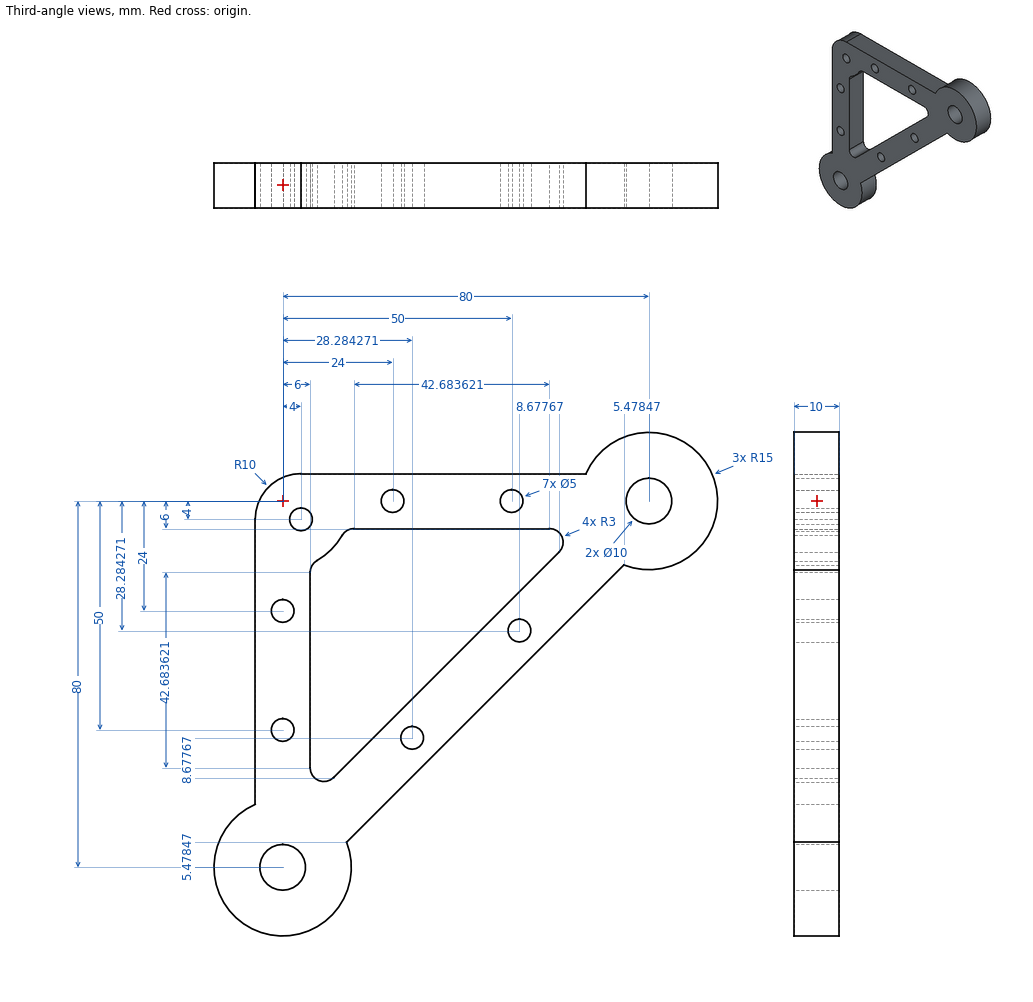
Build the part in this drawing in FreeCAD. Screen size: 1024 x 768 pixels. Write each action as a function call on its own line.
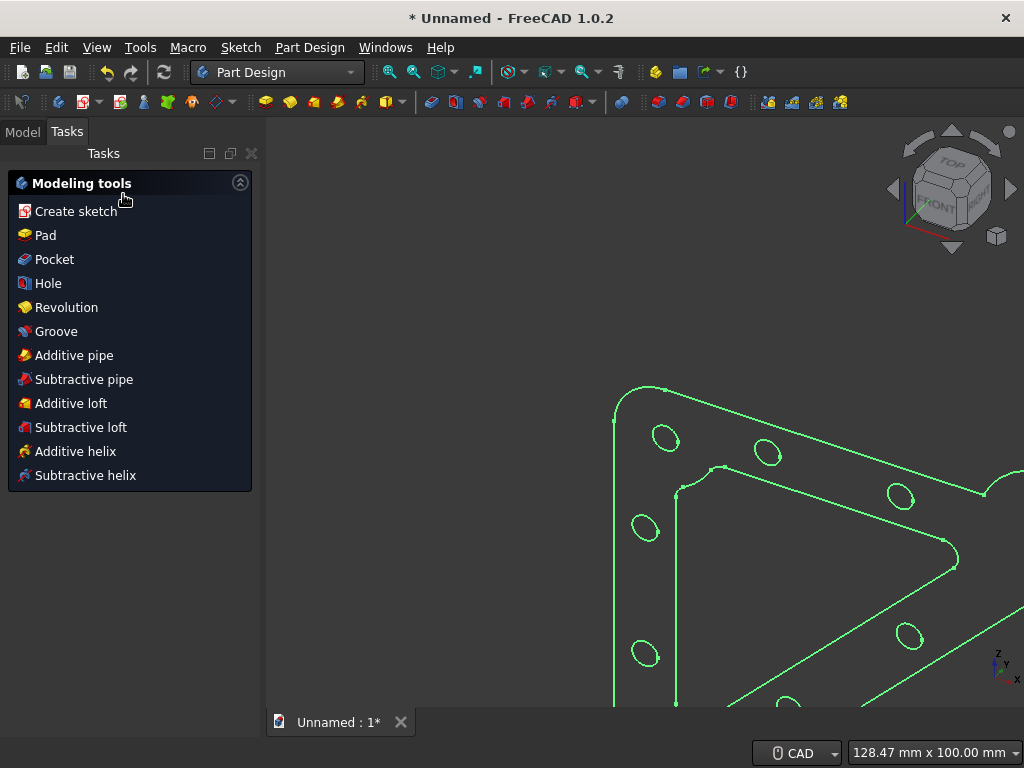
click(266, 102)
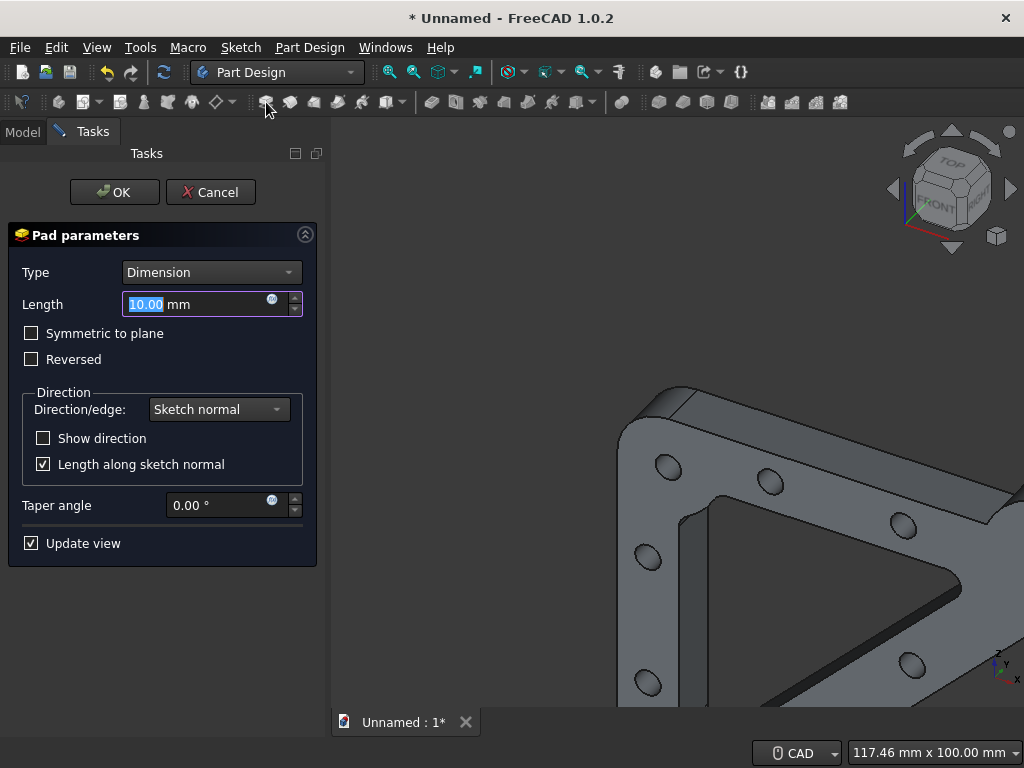
text(10)
key(Tab)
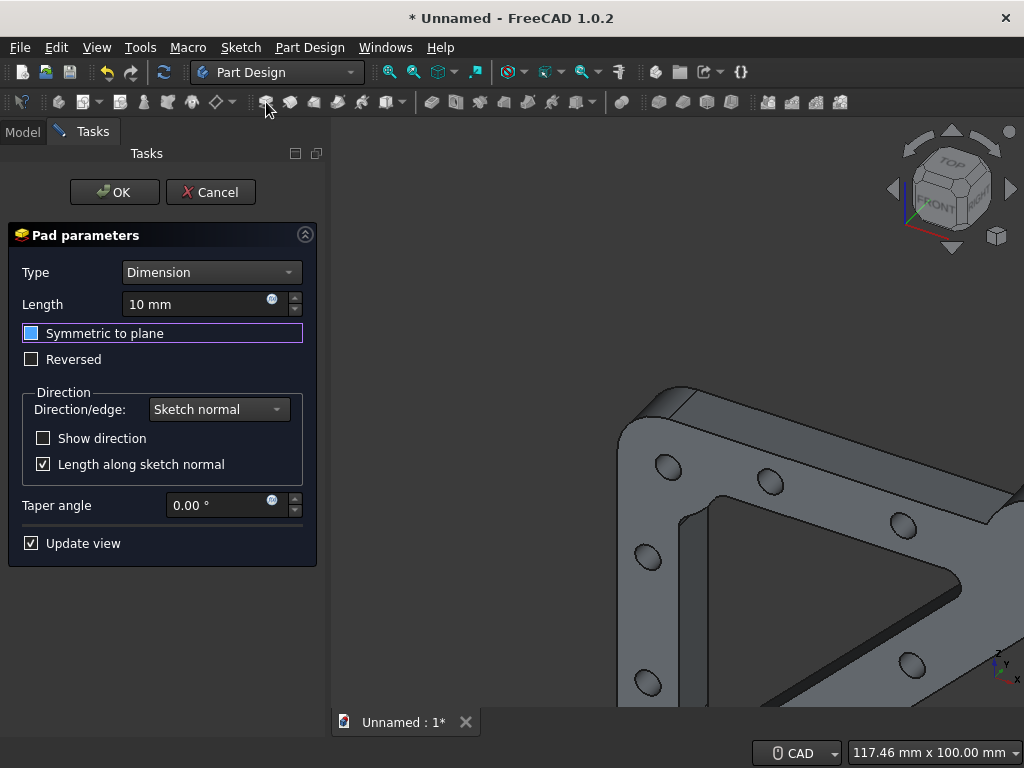
click(30, 333)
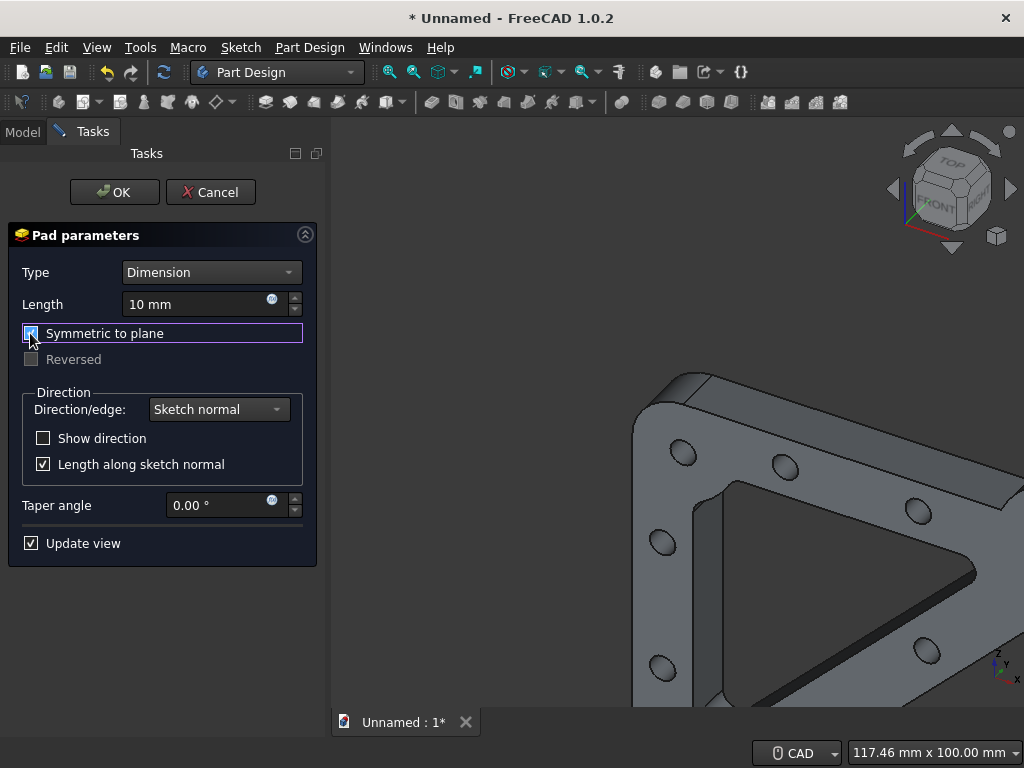
click(115, 192)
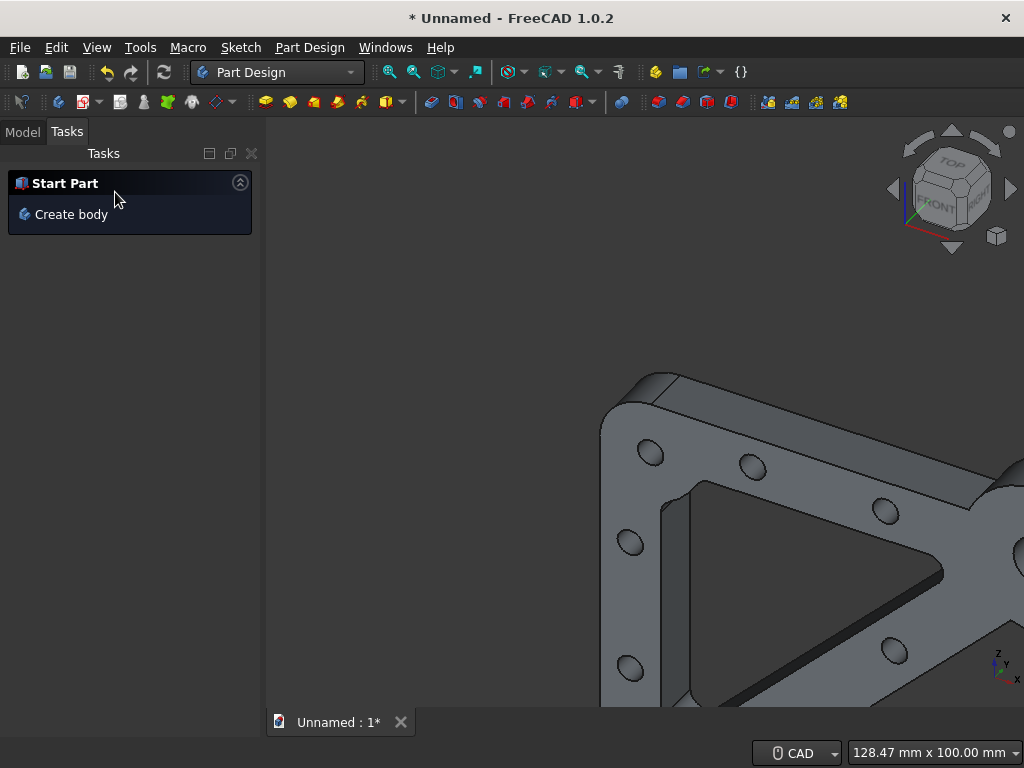
key(0)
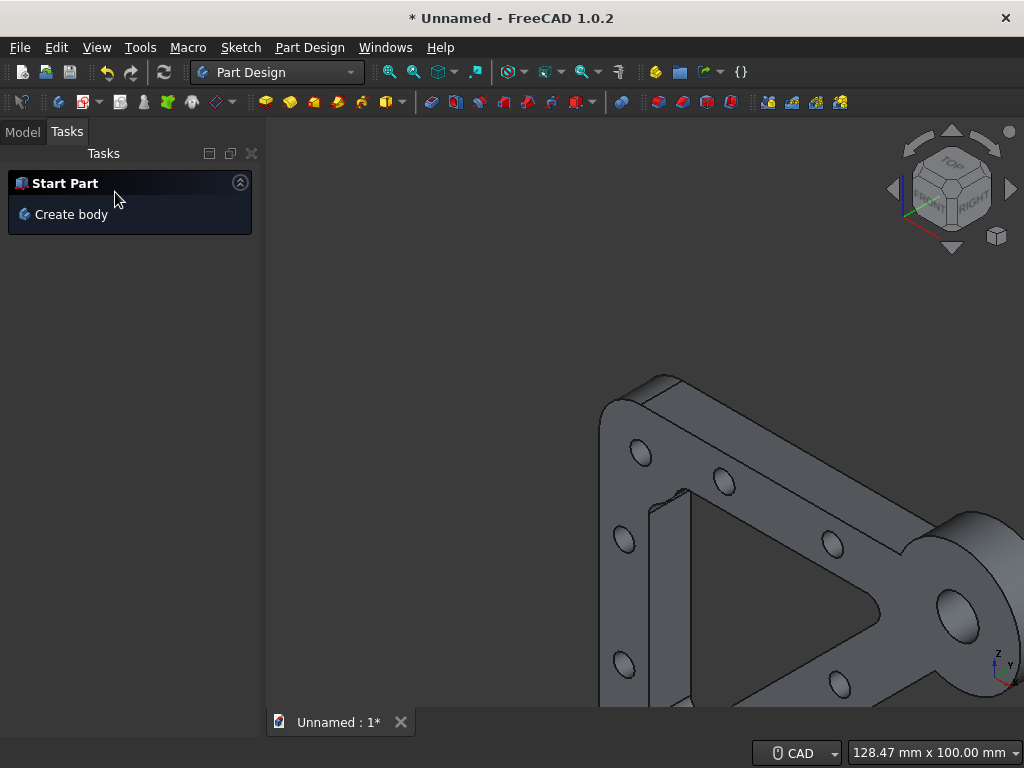
click(390, 72)